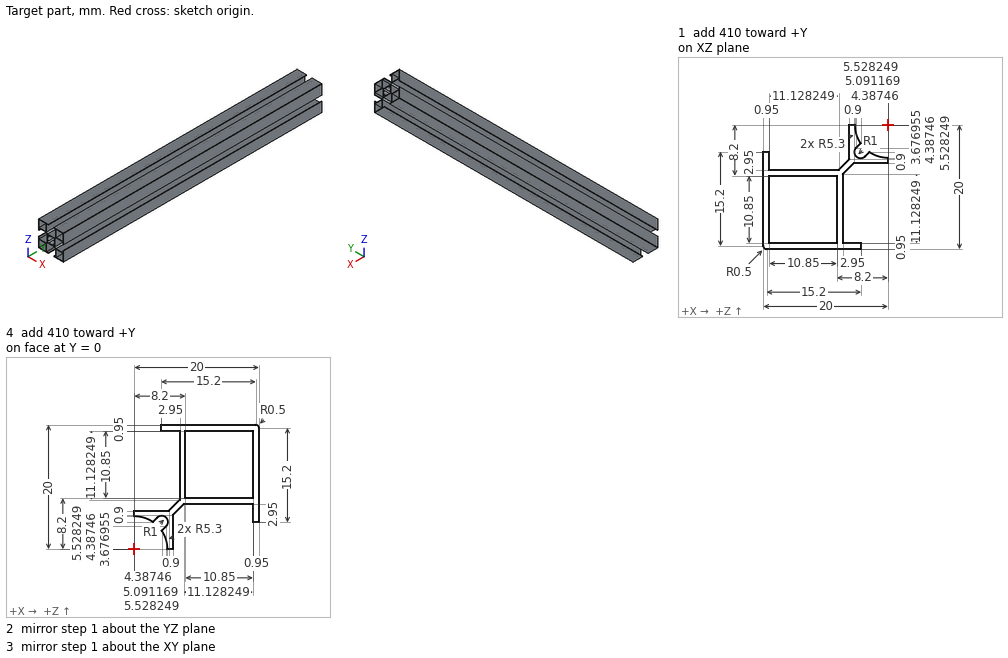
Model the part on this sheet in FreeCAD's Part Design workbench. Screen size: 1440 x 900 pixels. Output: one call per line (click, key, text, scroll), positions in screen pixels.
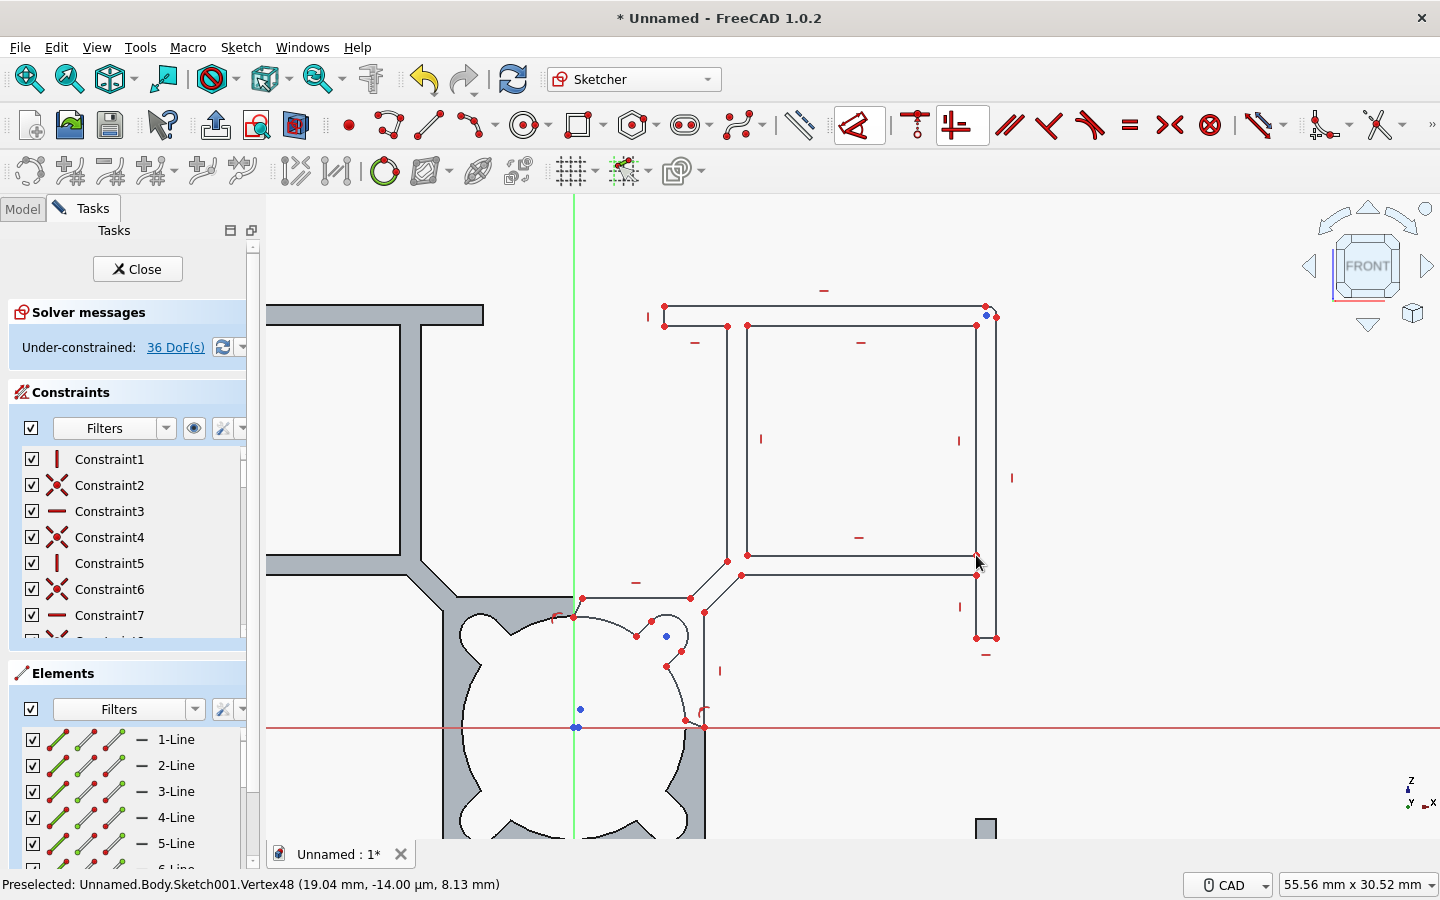
click(996, 414)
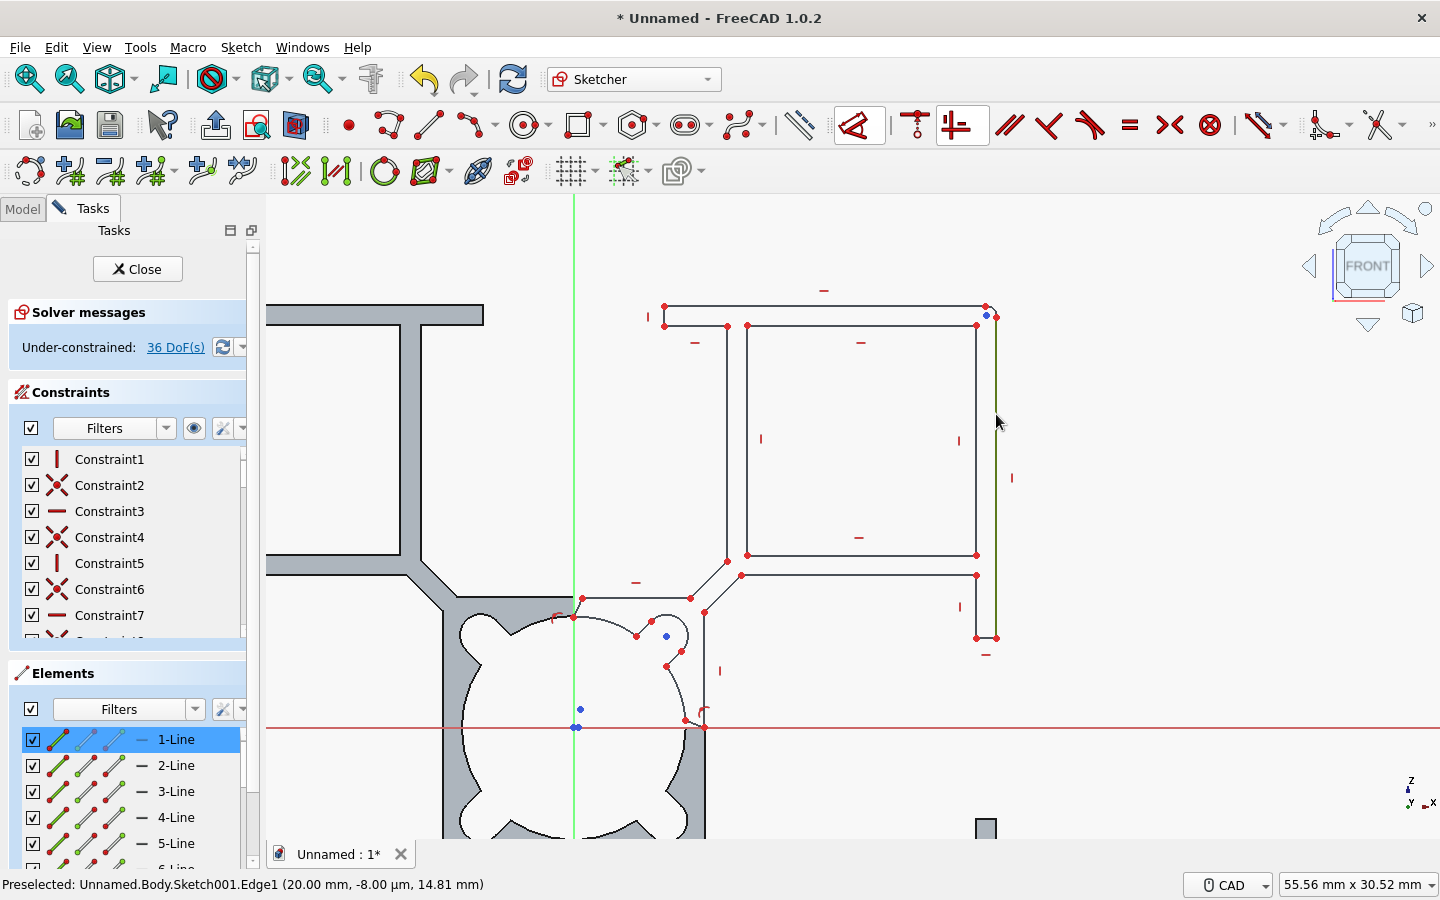
scroll(994, 309, up, 3)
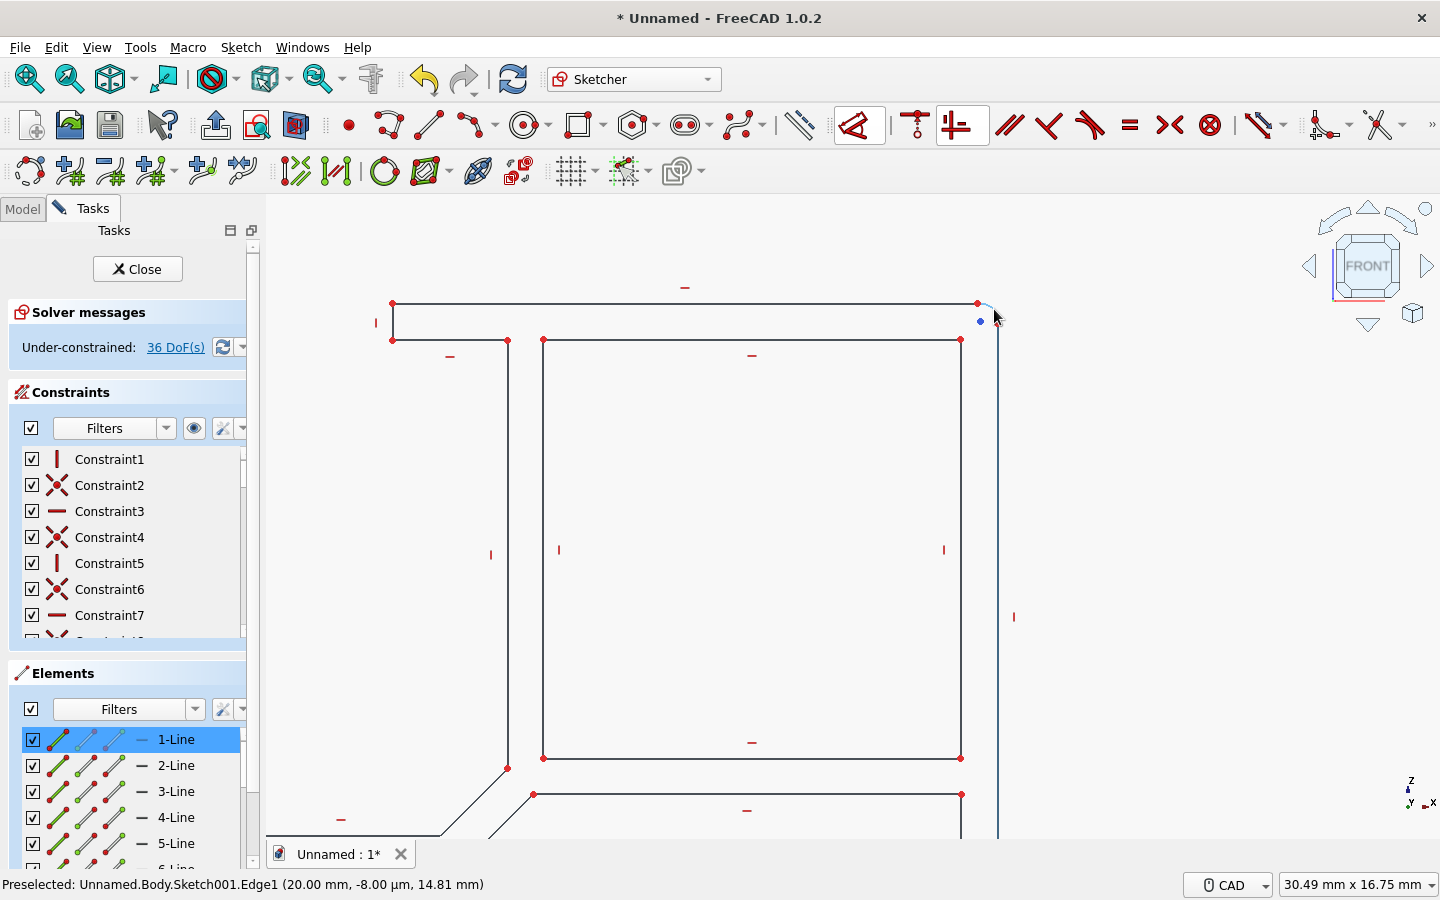
click(993, 309)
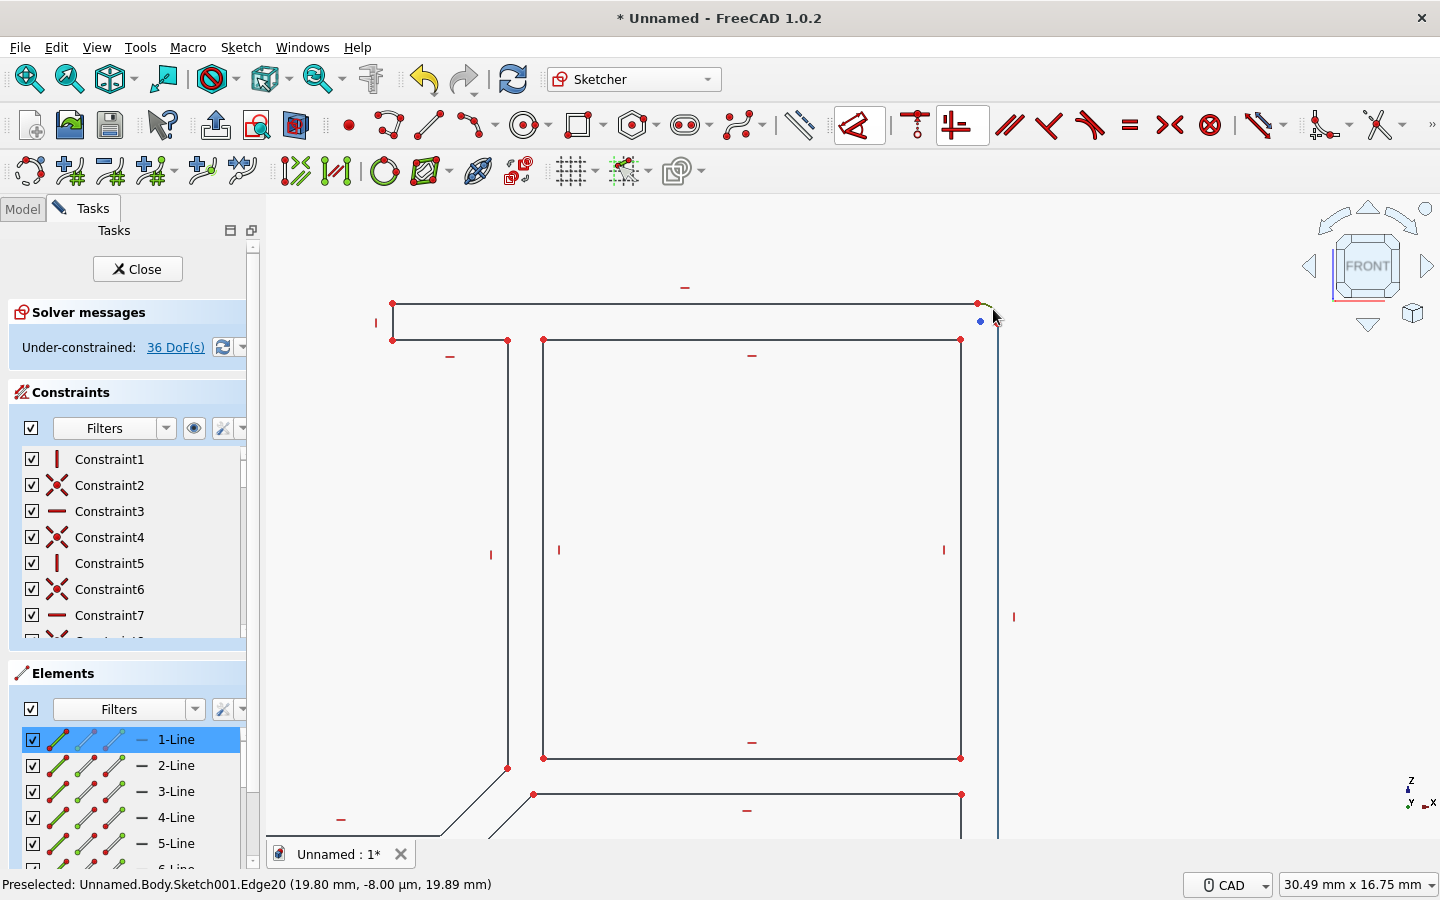
click(1090, 126)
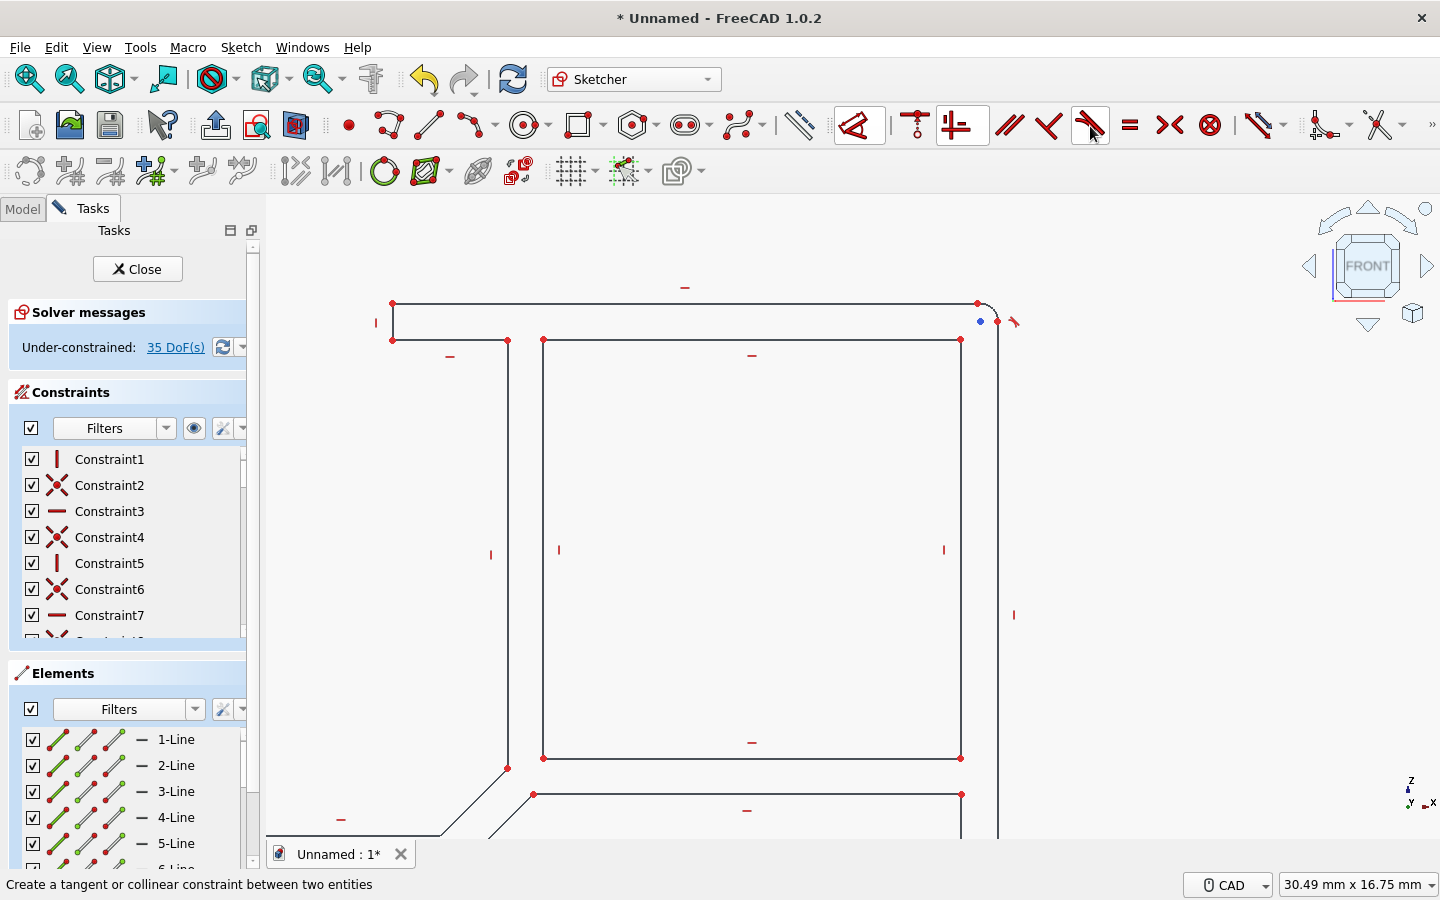
scroll(993, 309, down, 3)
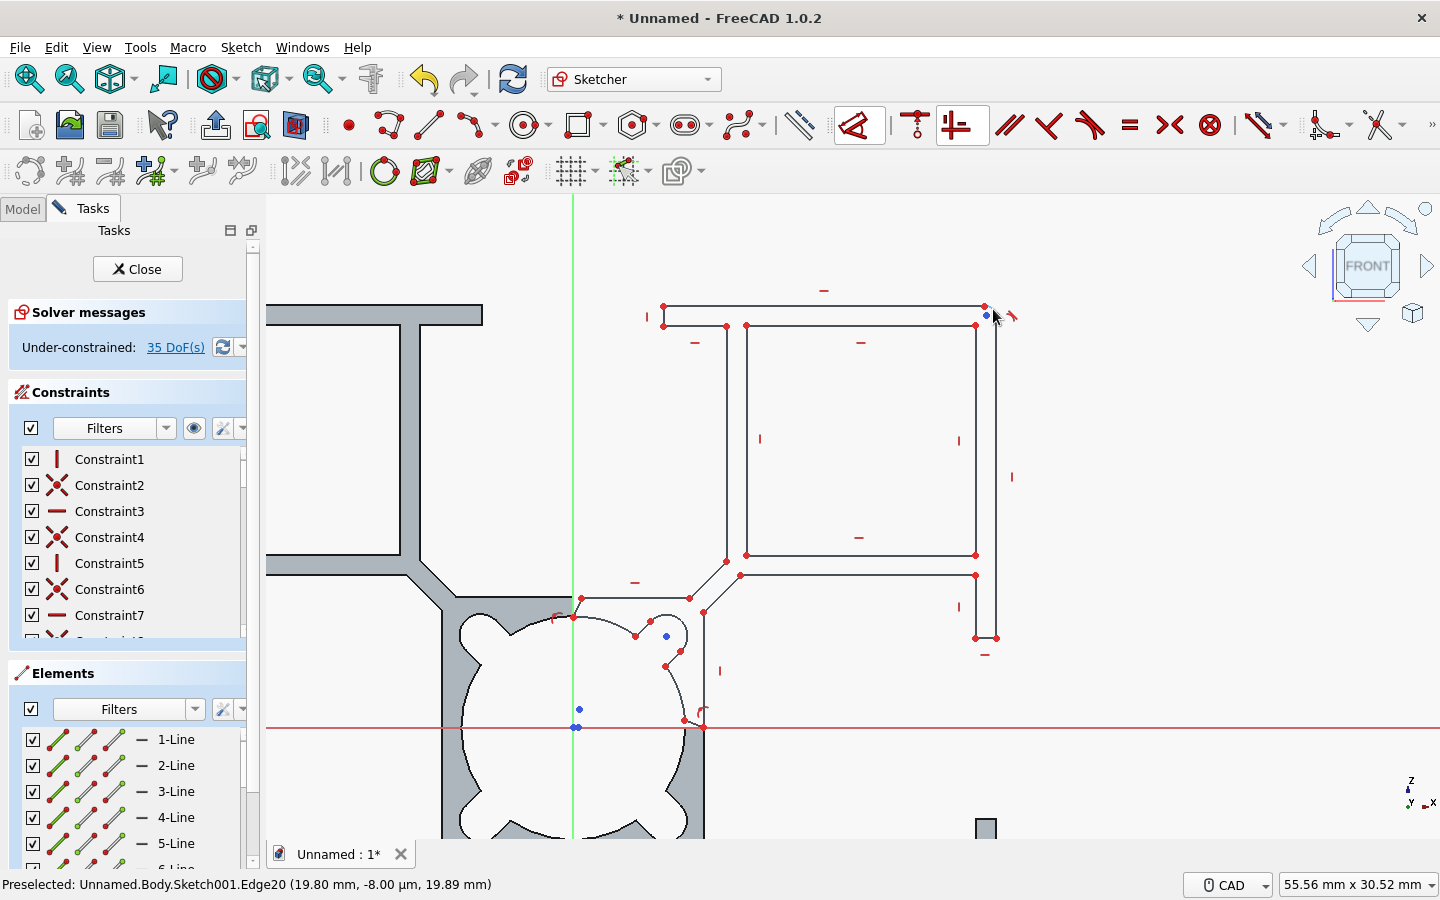
scroll(670, 662, up, 4)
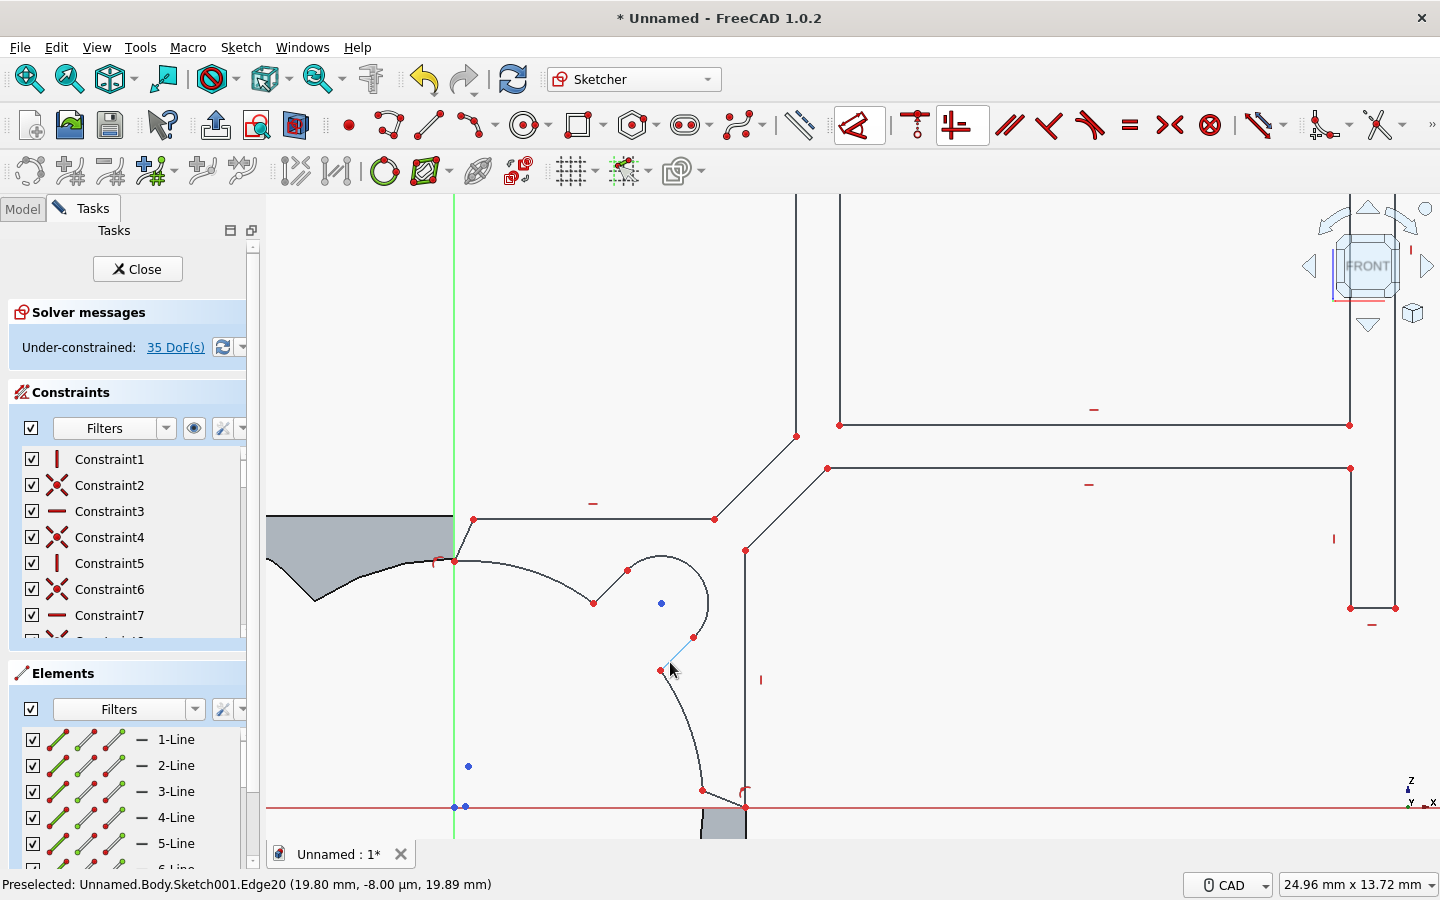
click(671, 661)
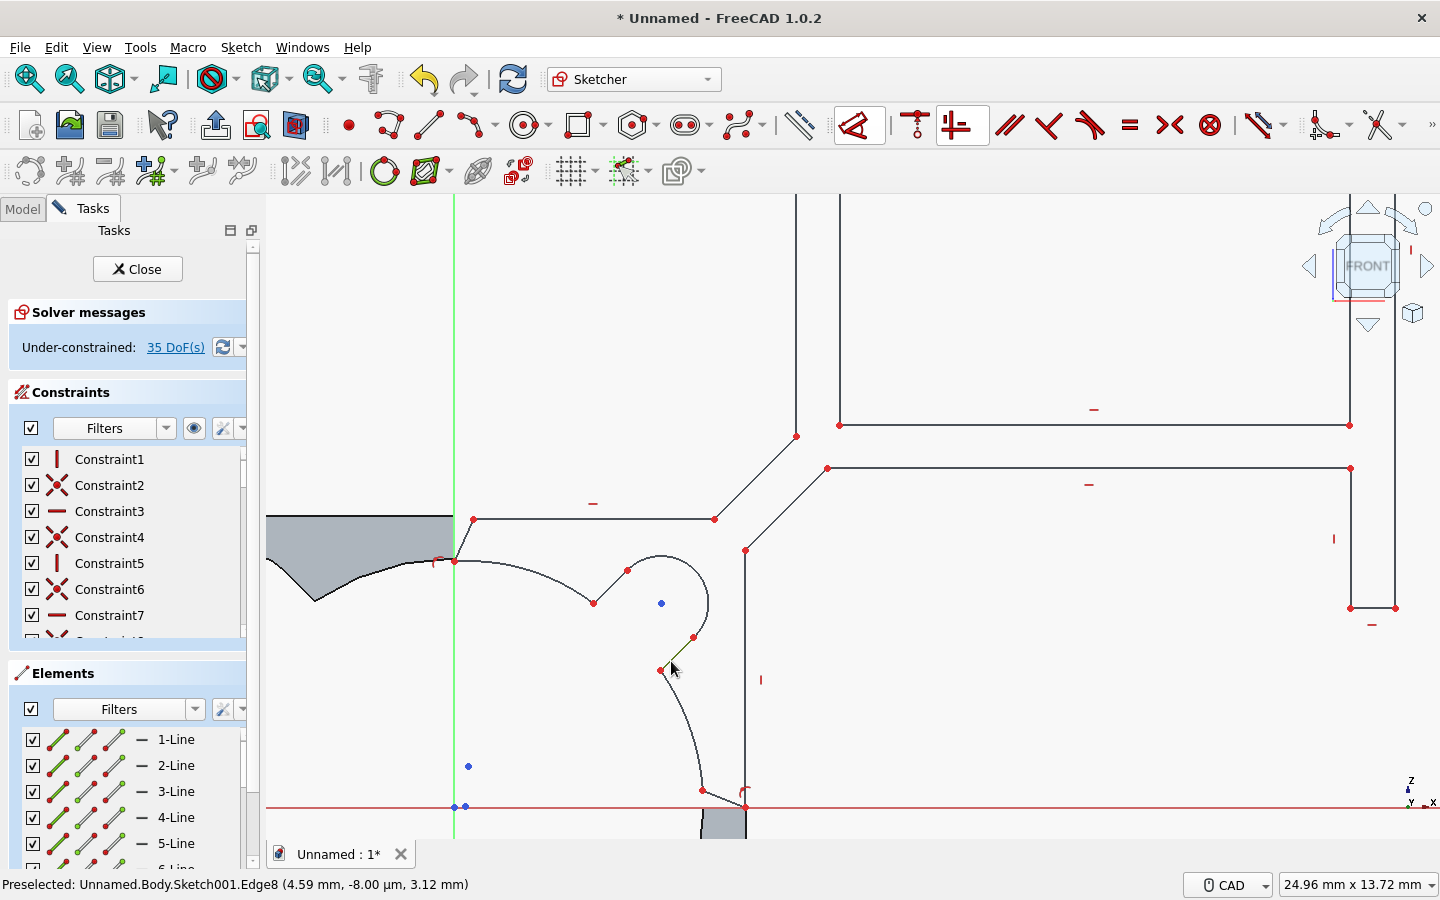
click(708, 596)